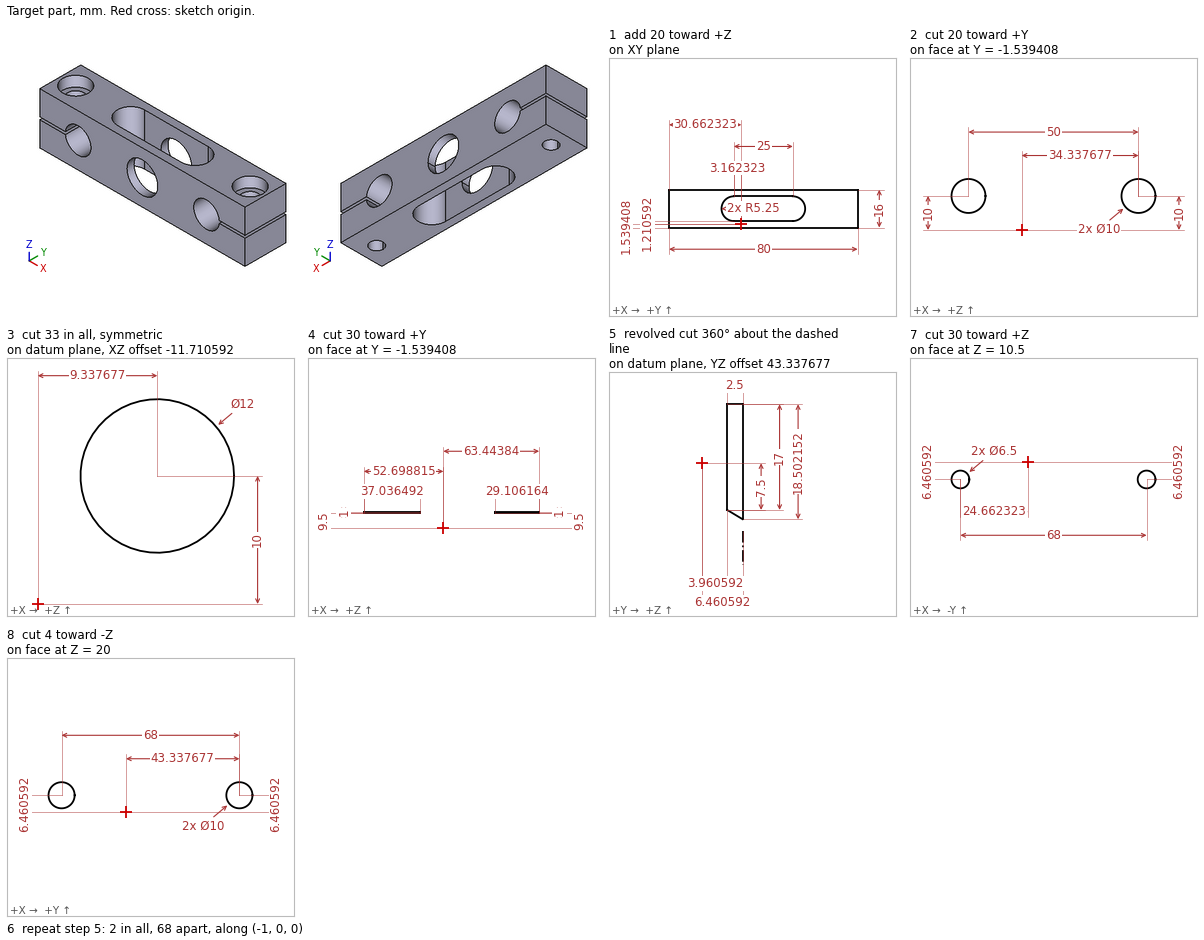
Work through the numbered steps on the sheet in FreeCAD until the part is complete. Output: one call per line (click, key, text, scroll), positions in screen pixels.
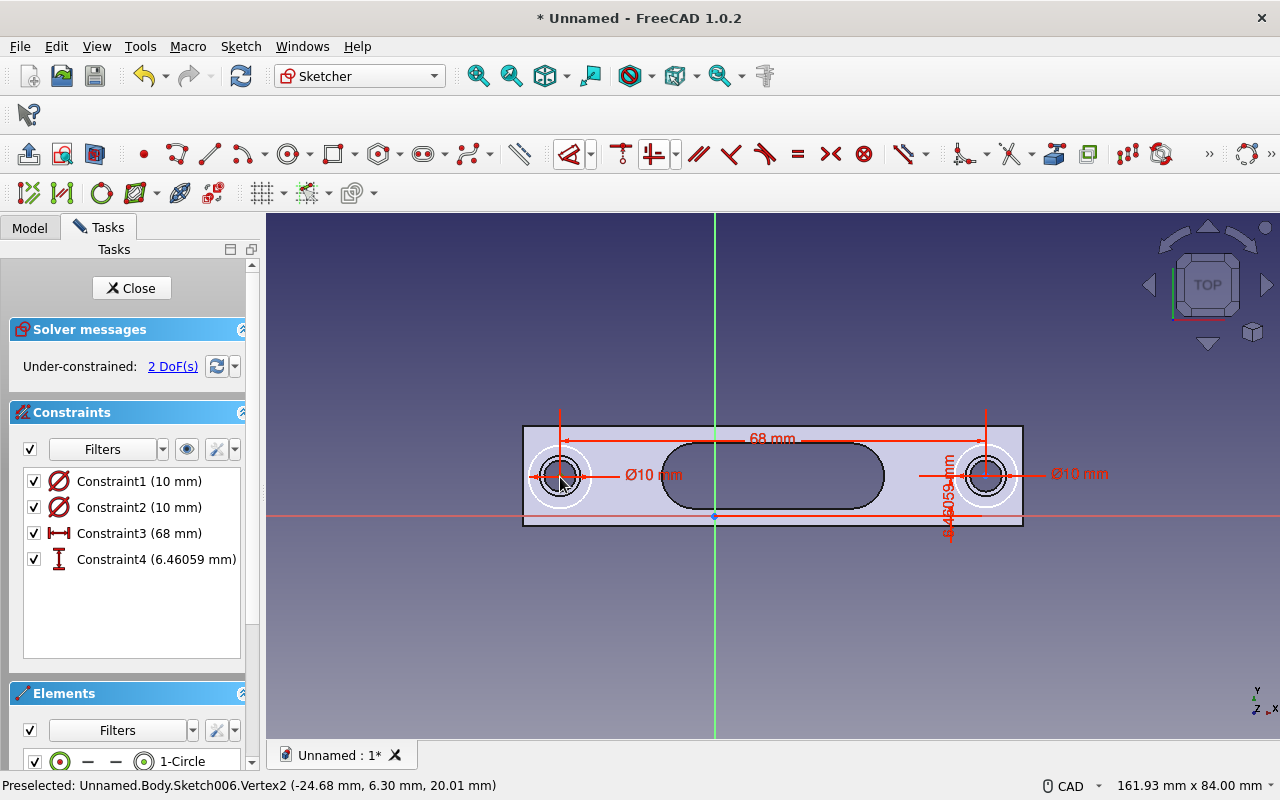
key(i)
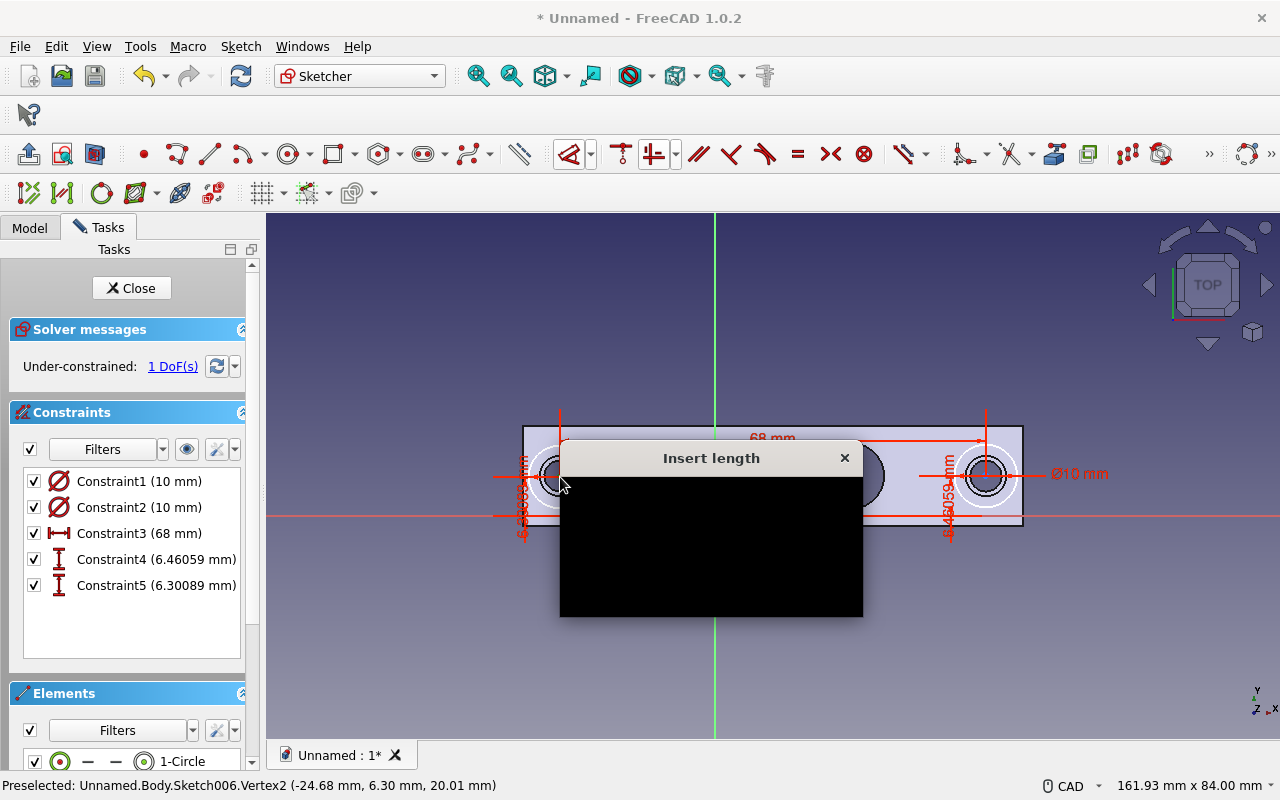
text(6.460592)
key(Return)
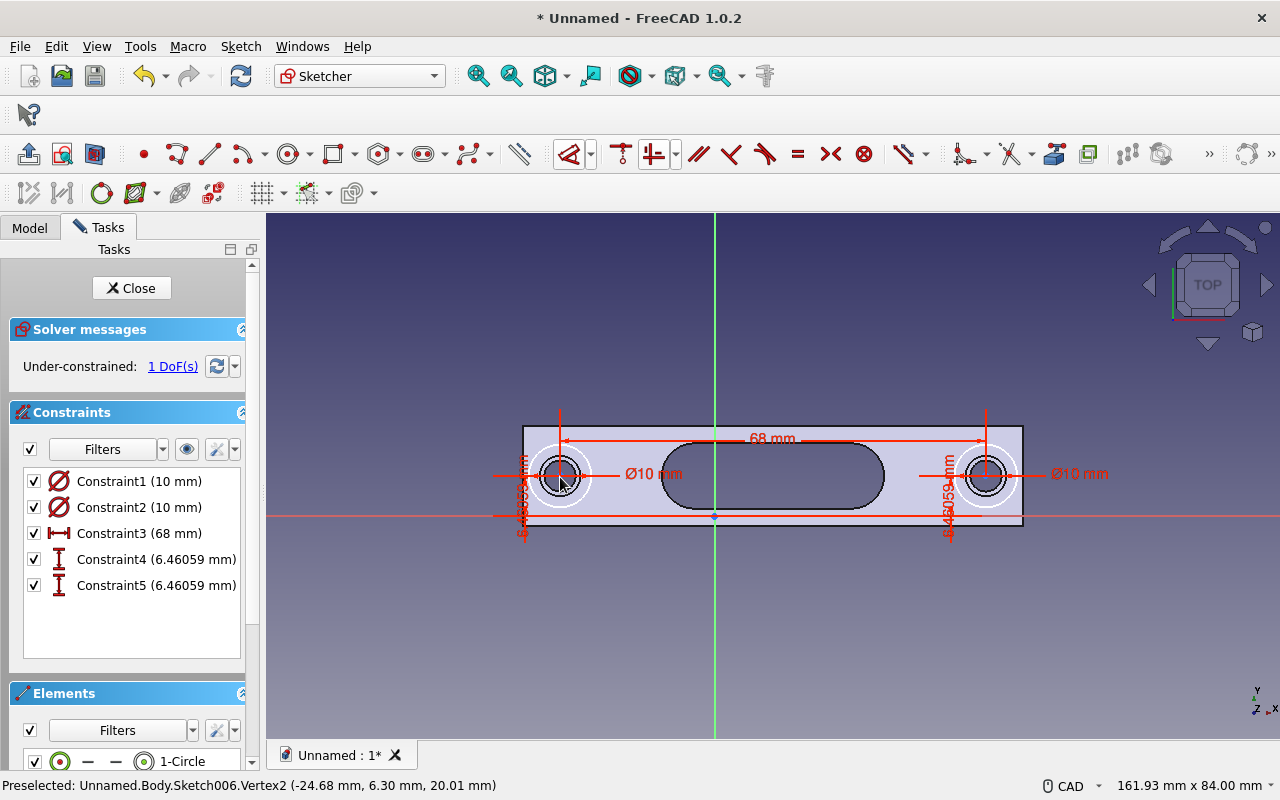
click(986, 476)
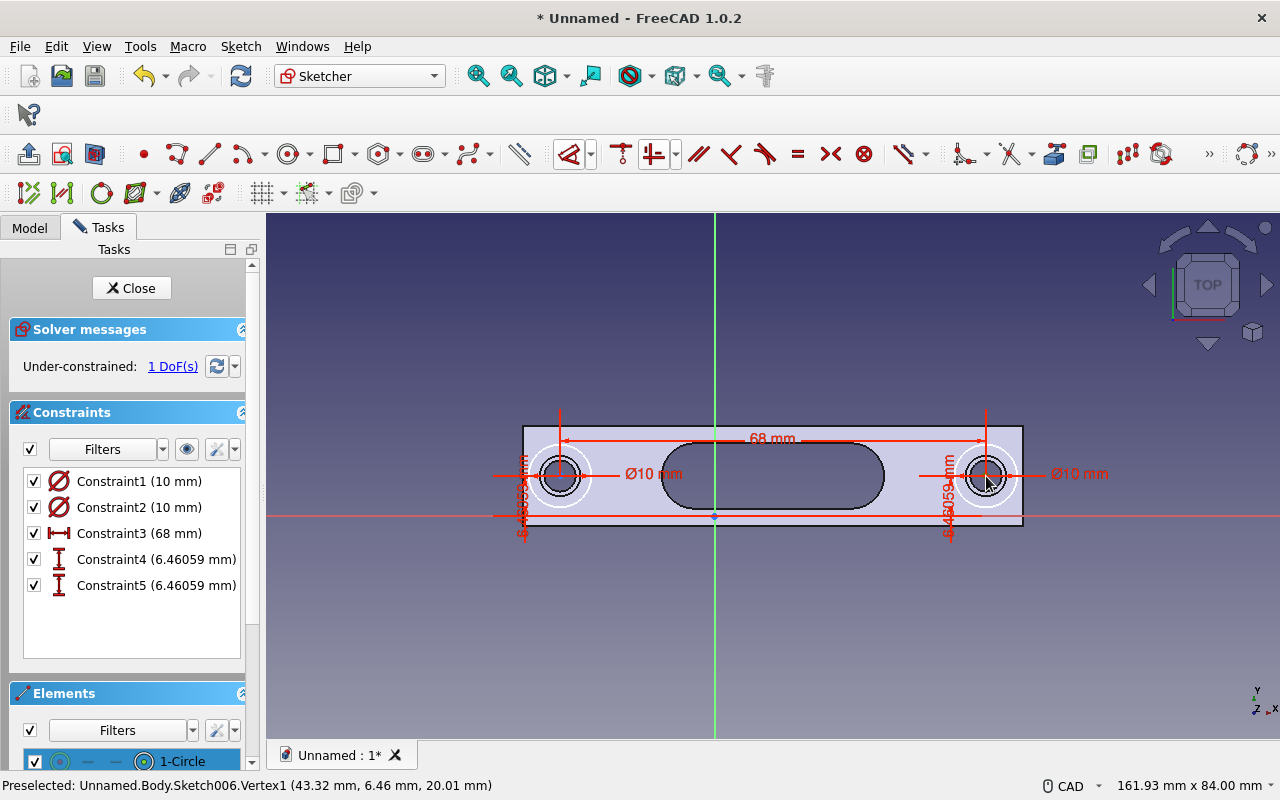
key(l)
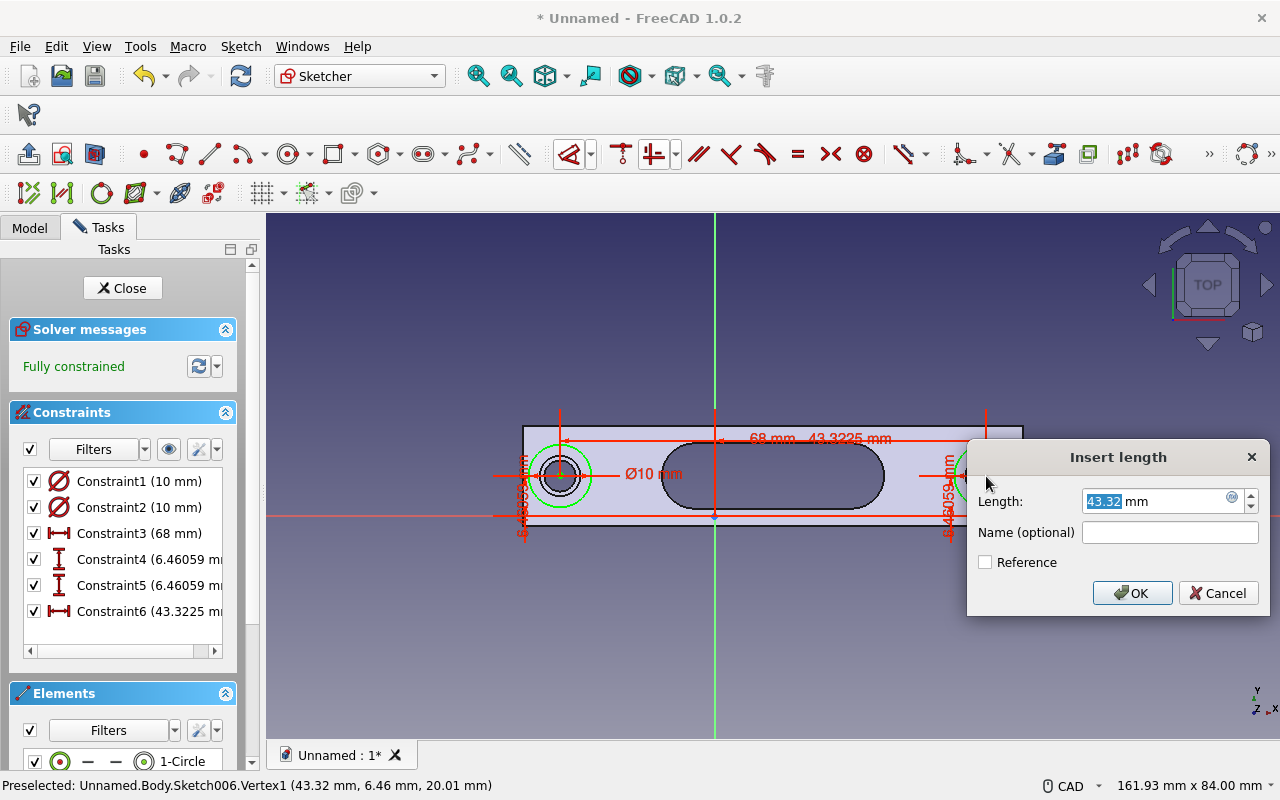
text(43.337677)
key(Return)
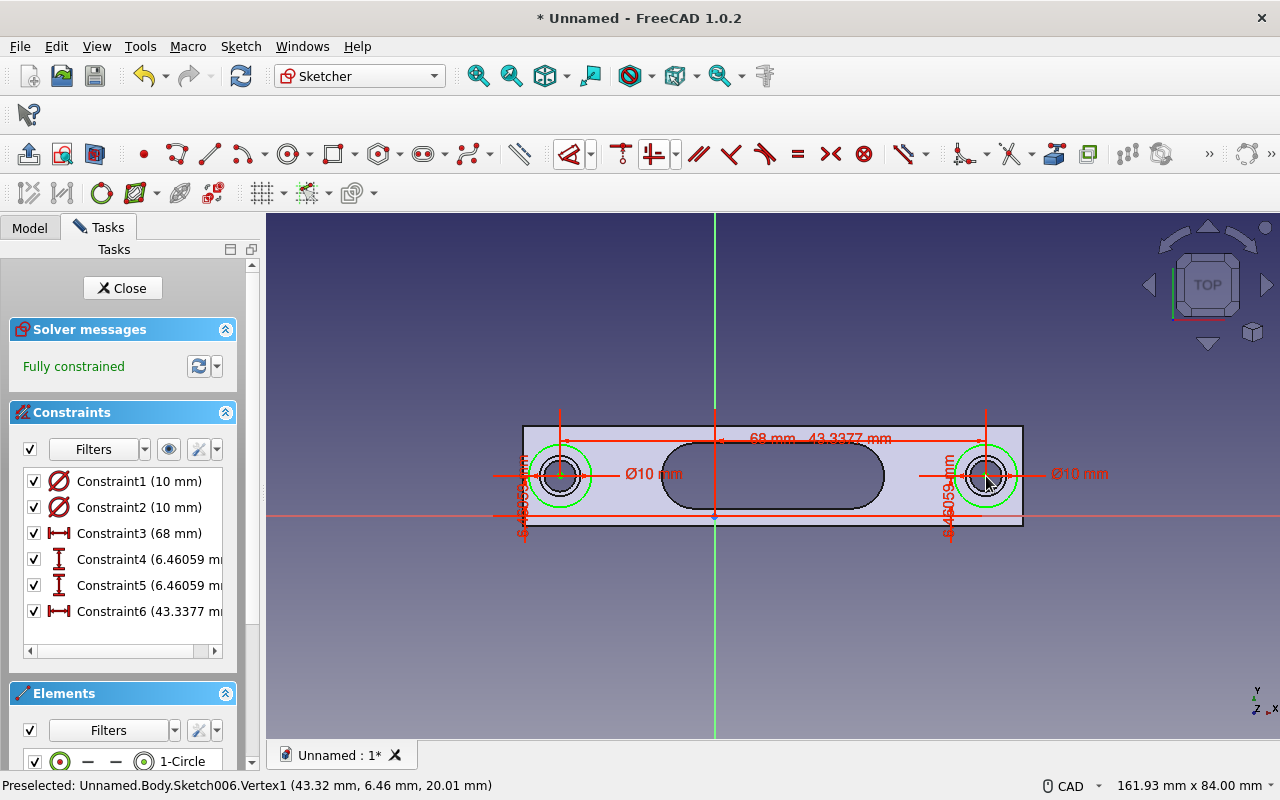
click(123, 288)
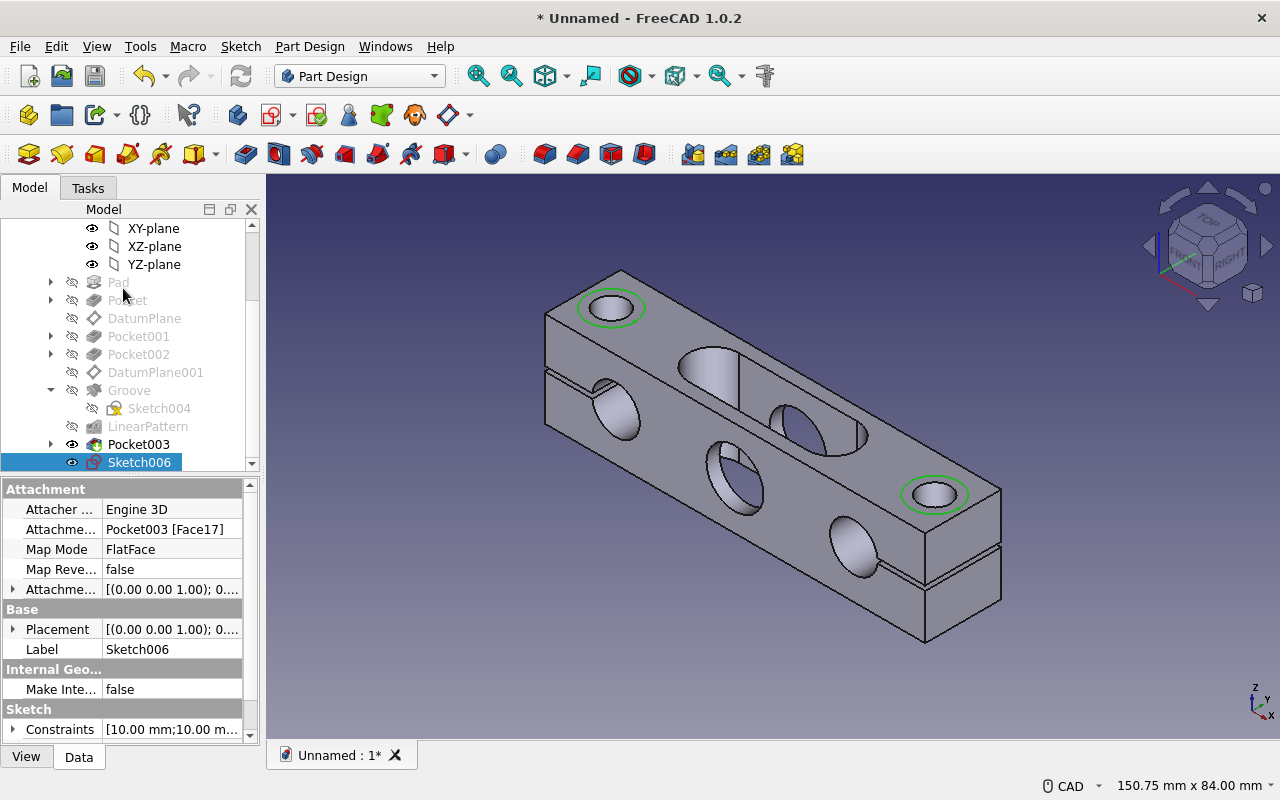
click(246, 154)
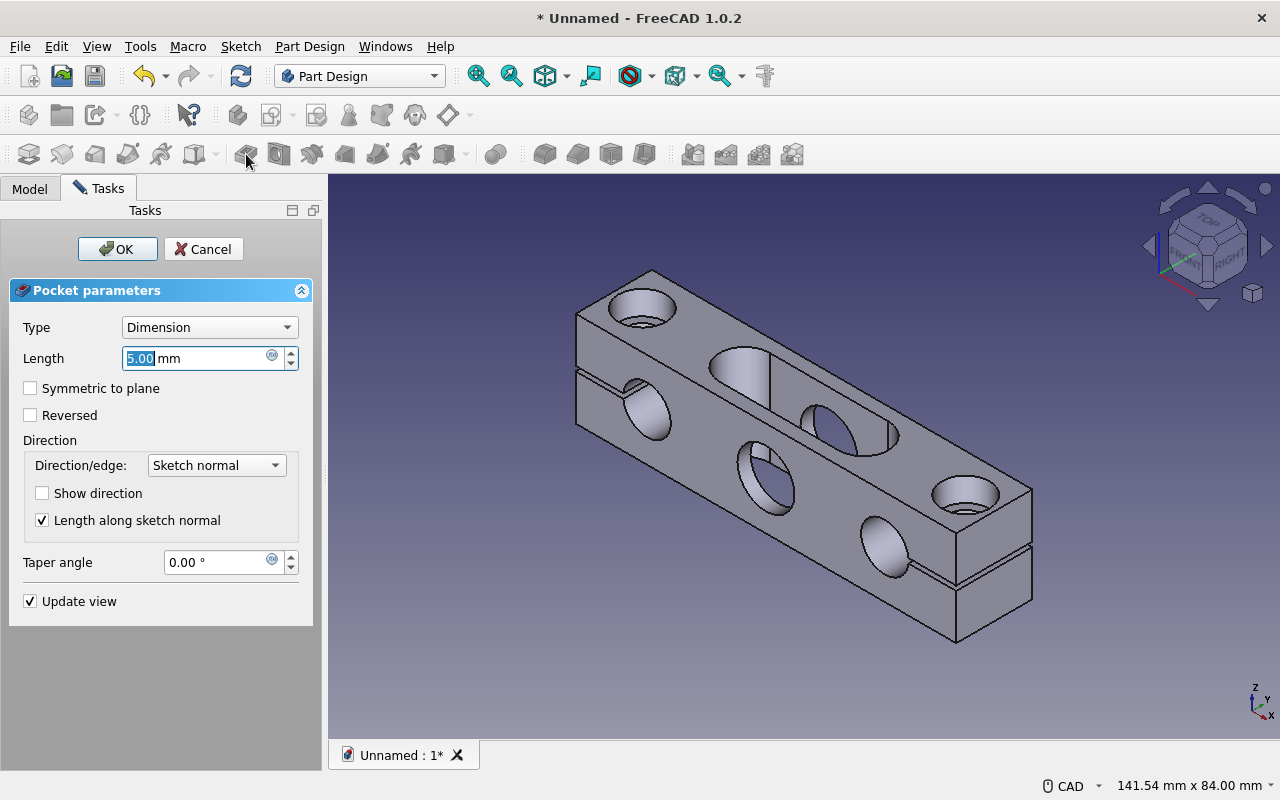
text(4)
key(Tab)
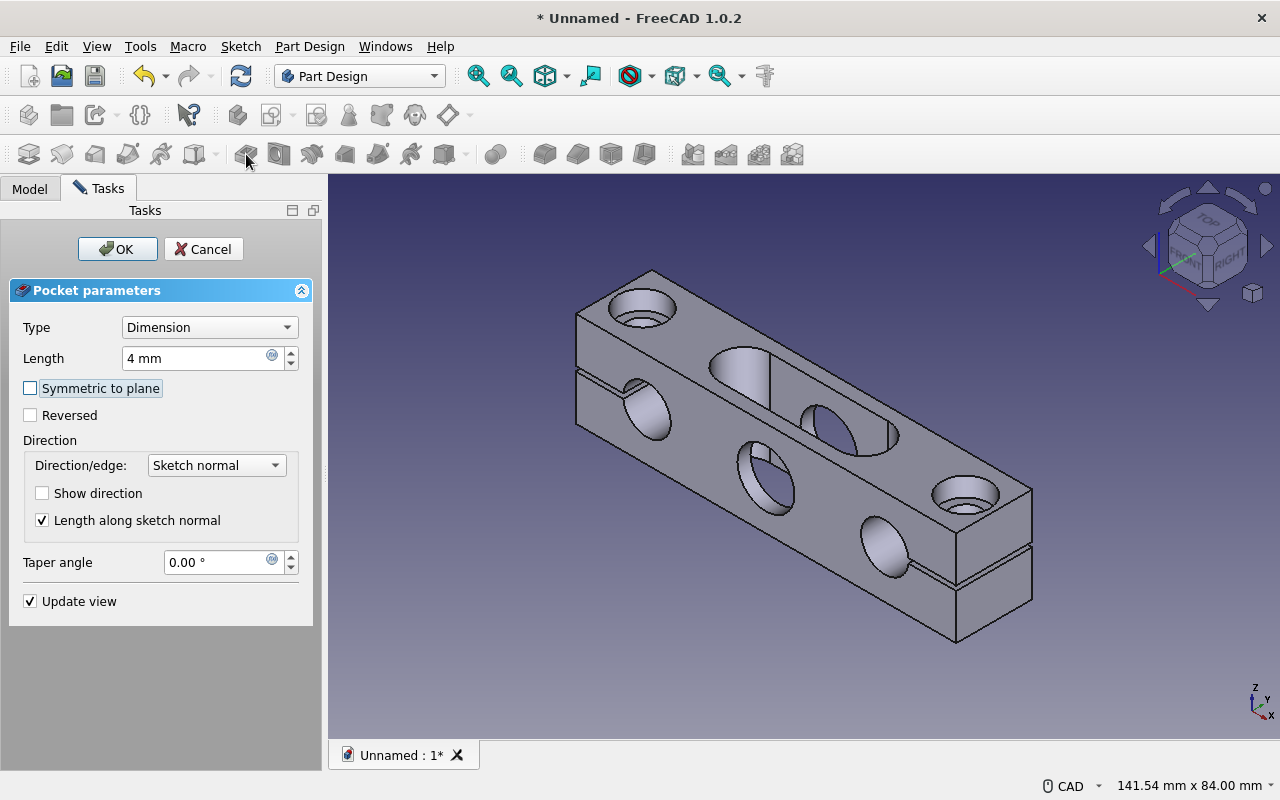
click(118, 249)